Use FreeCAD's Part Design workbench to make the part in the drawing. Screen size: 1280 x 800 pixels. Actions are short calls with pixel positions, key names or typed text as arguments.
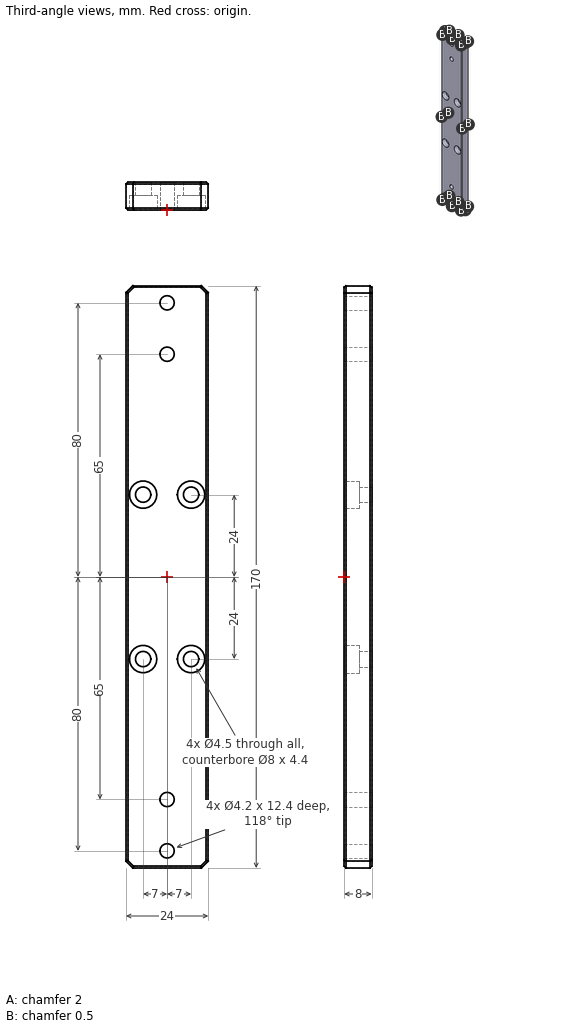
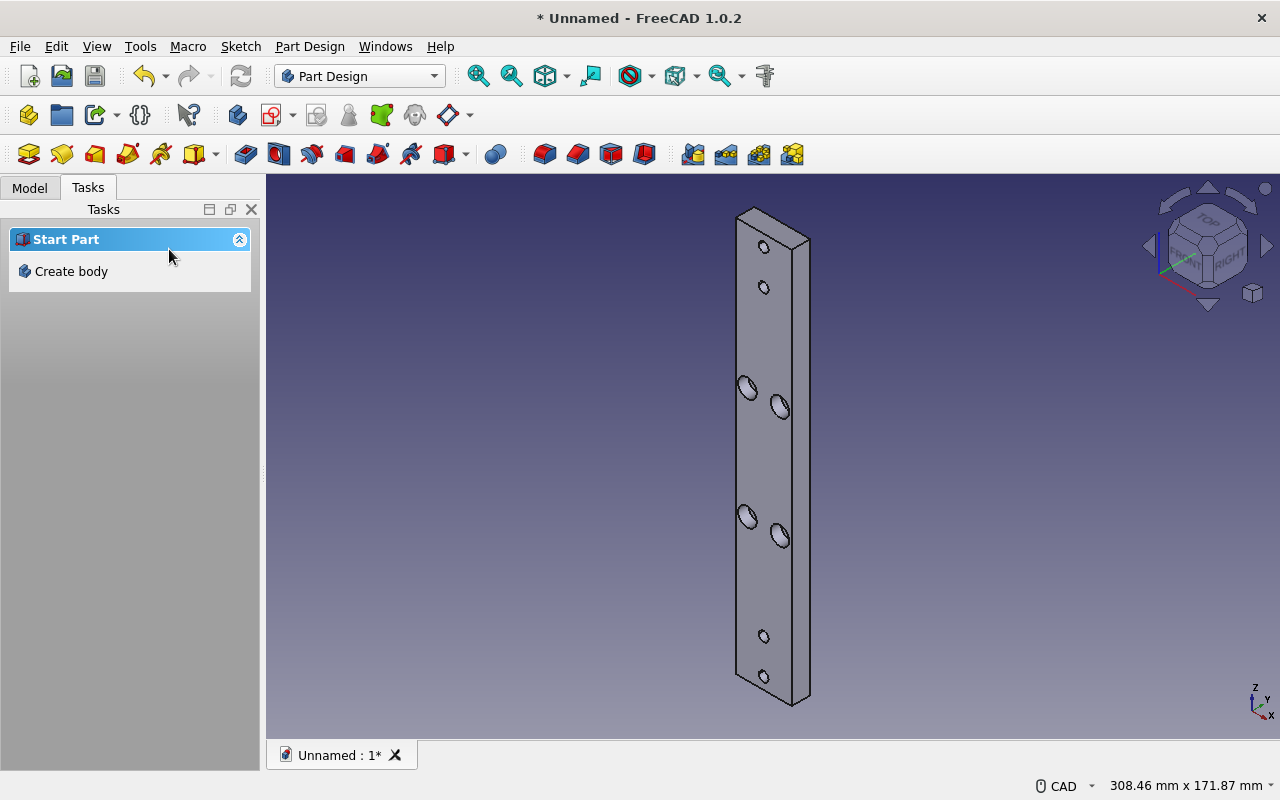
click(801, 243)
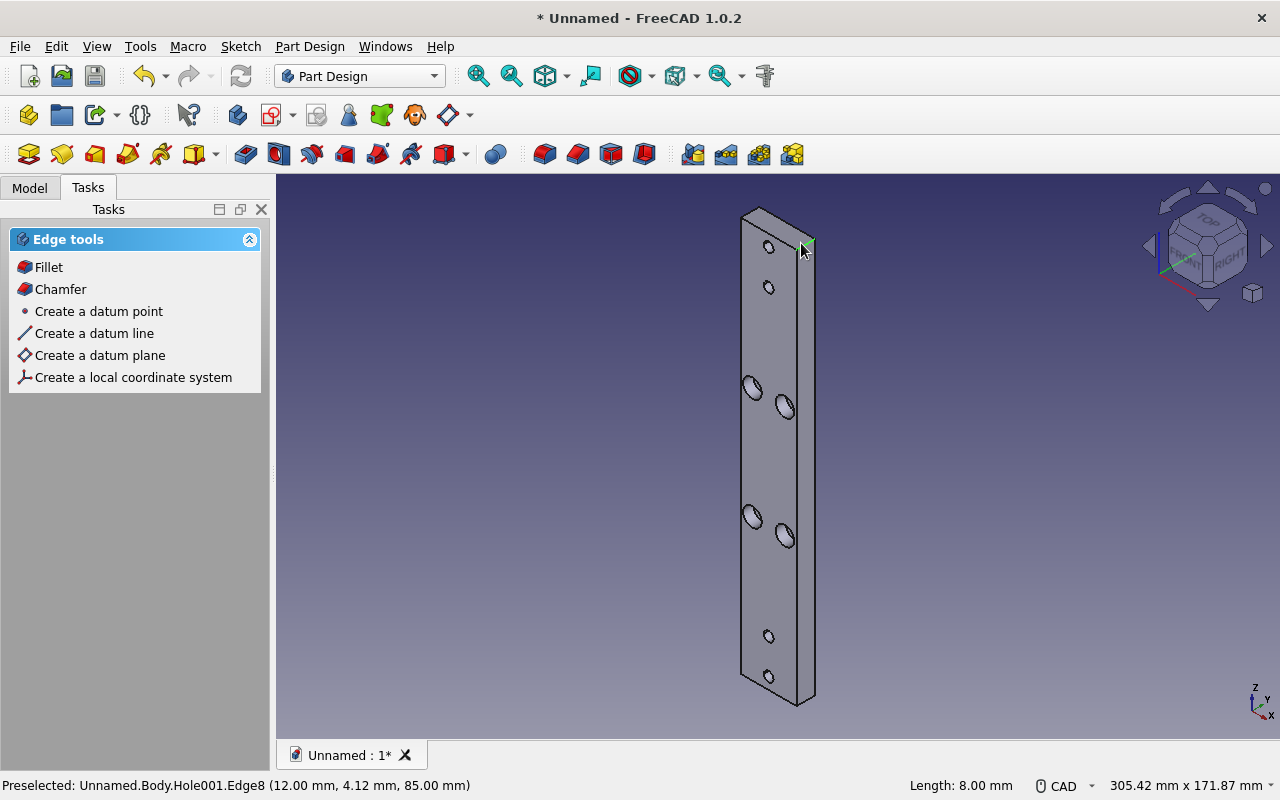
key(2)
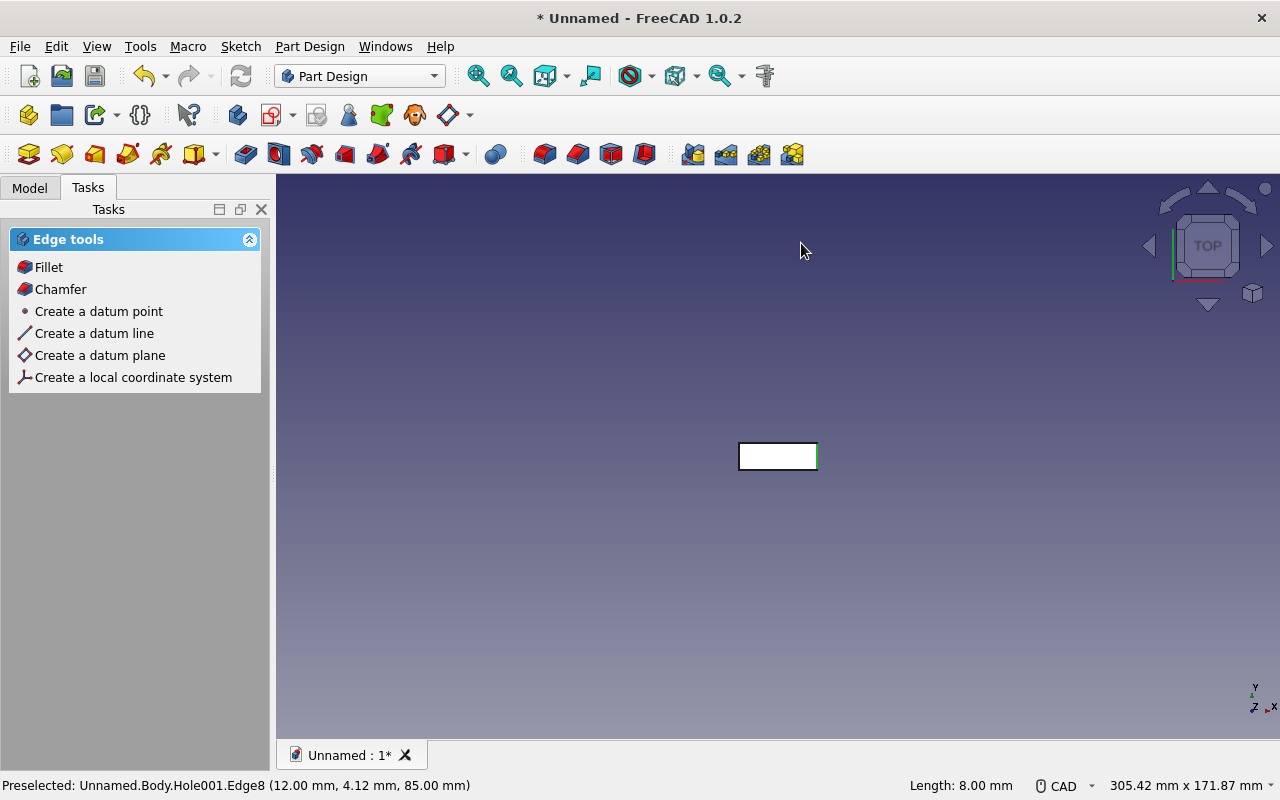
key(v)
key(f)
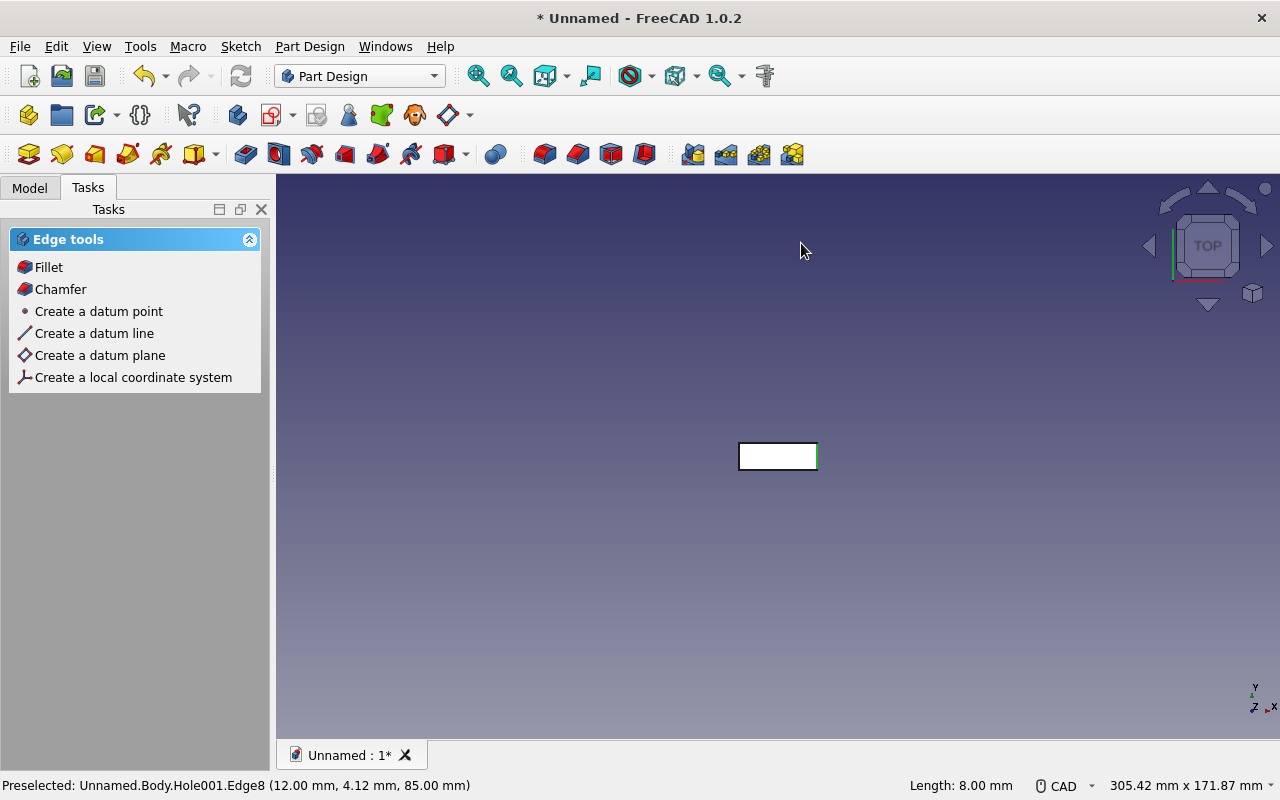
click(739, 455, ctrl)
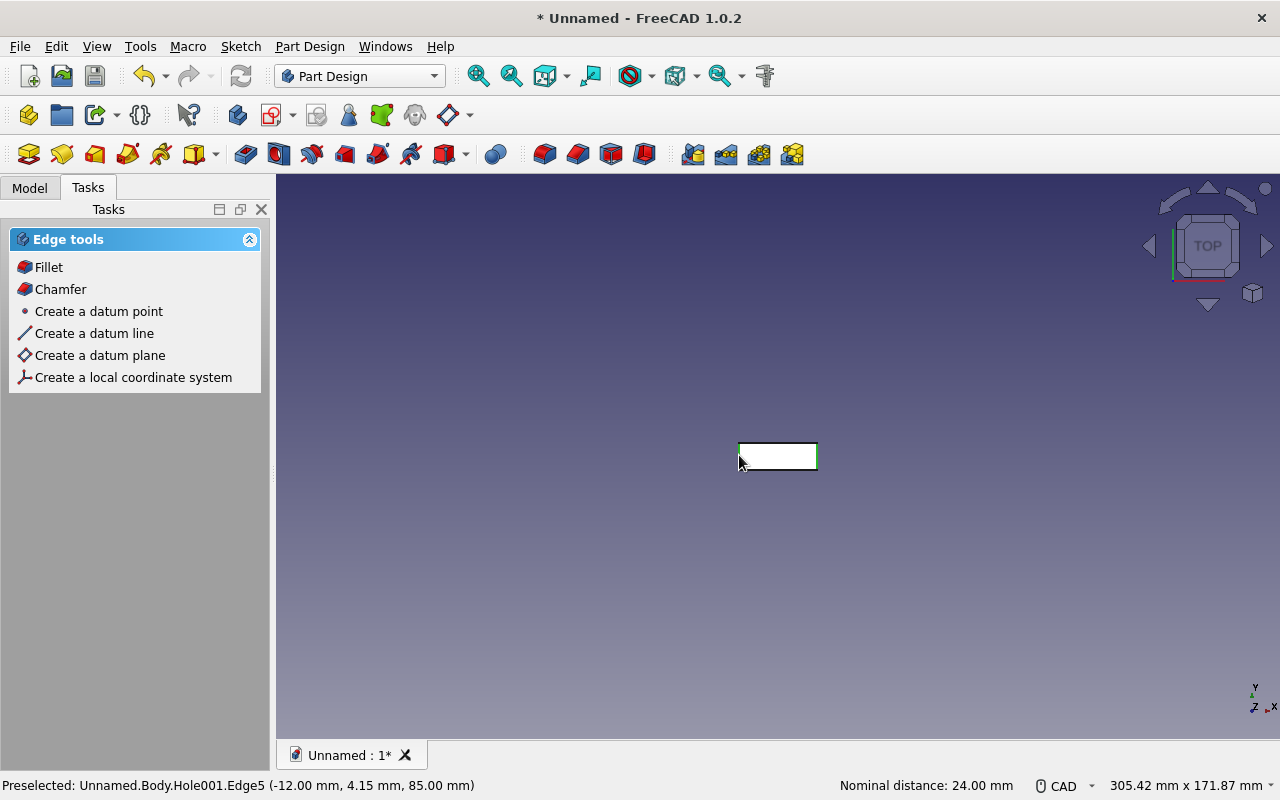
key(1)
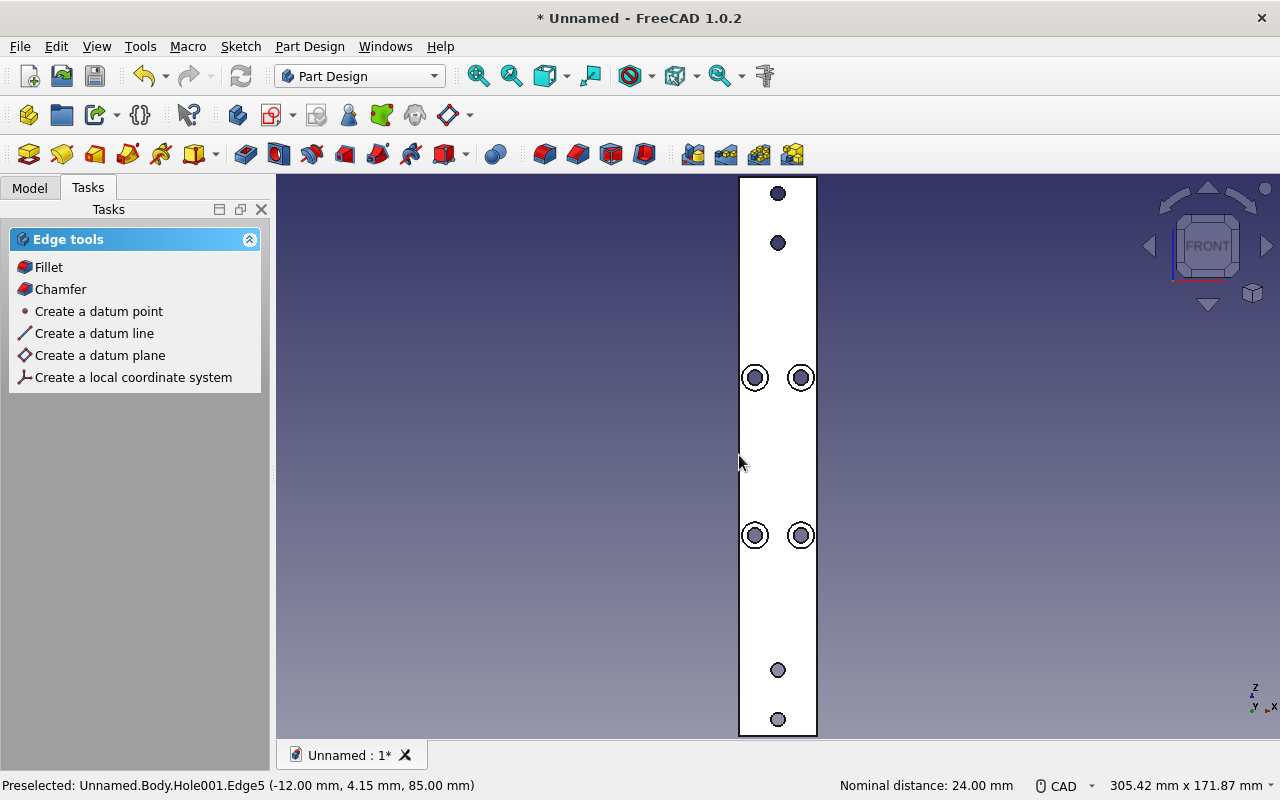
key(3)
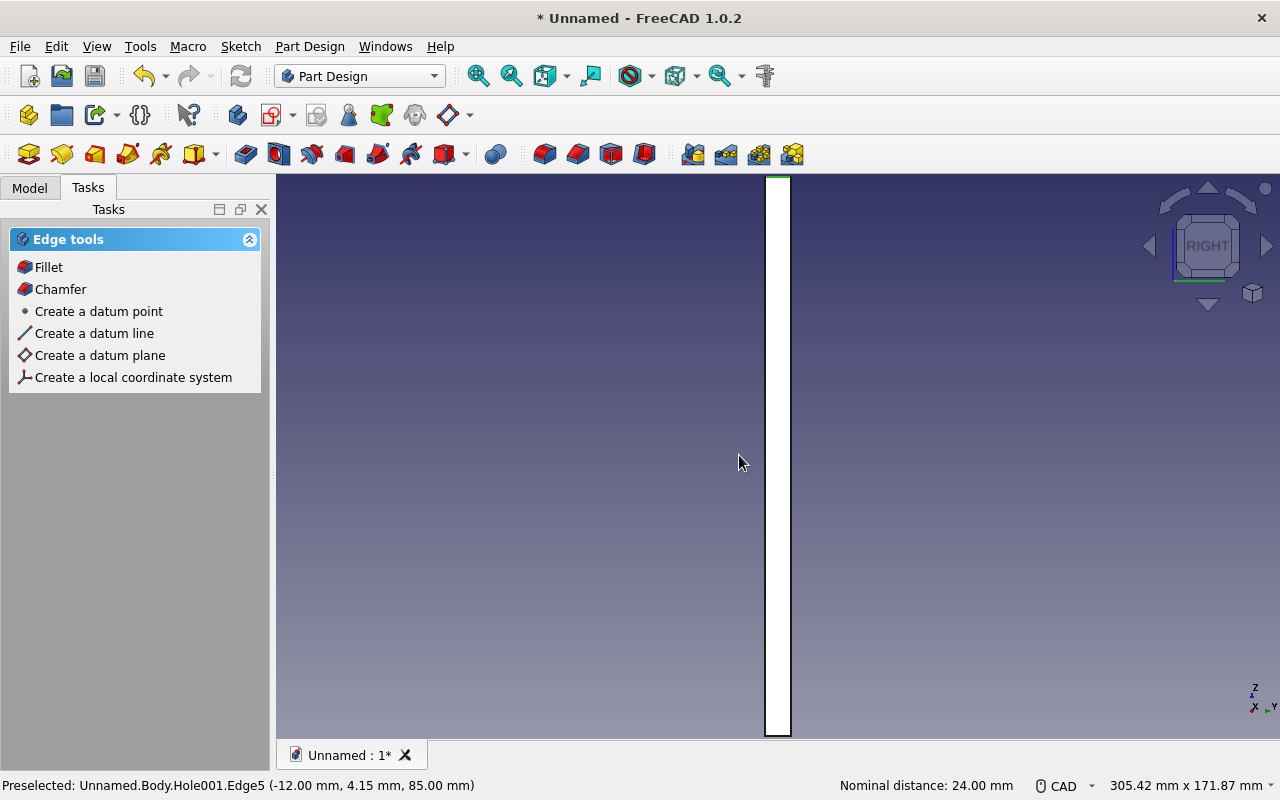
key(5)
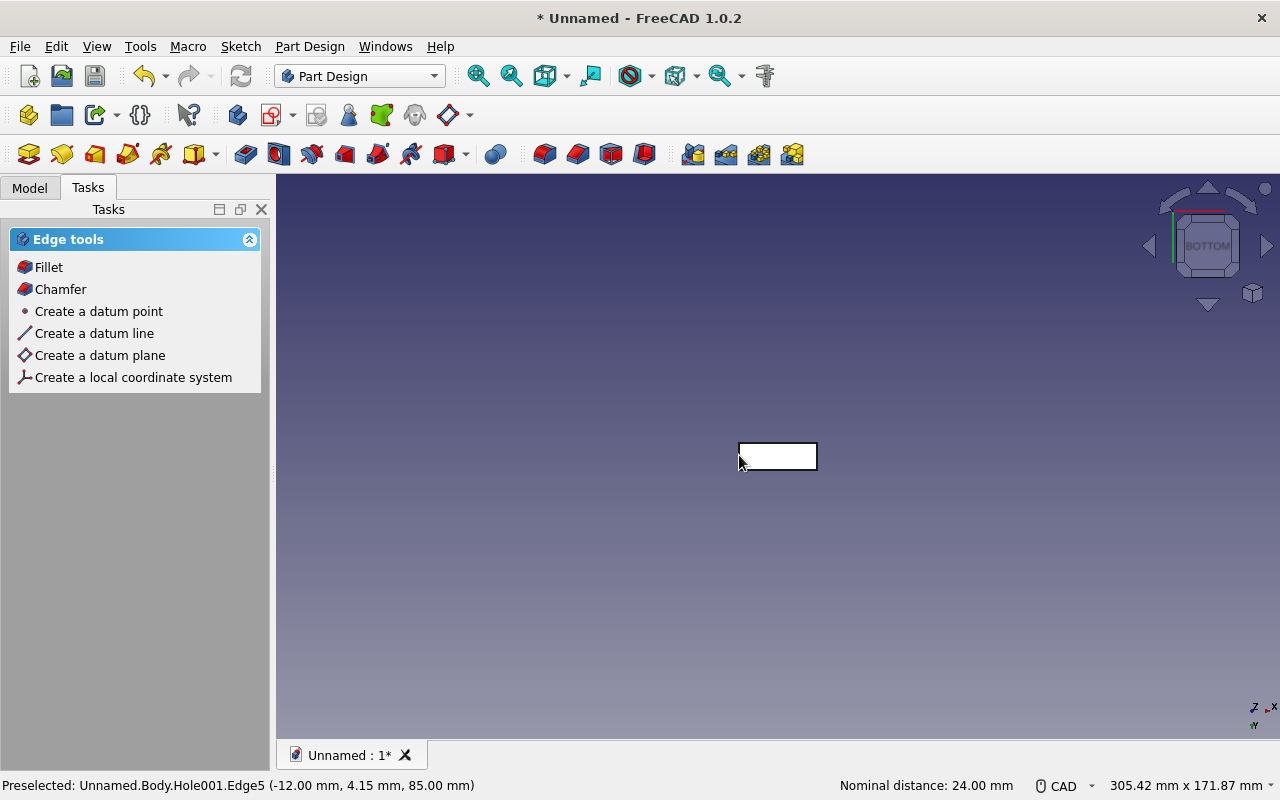
click(479, 76)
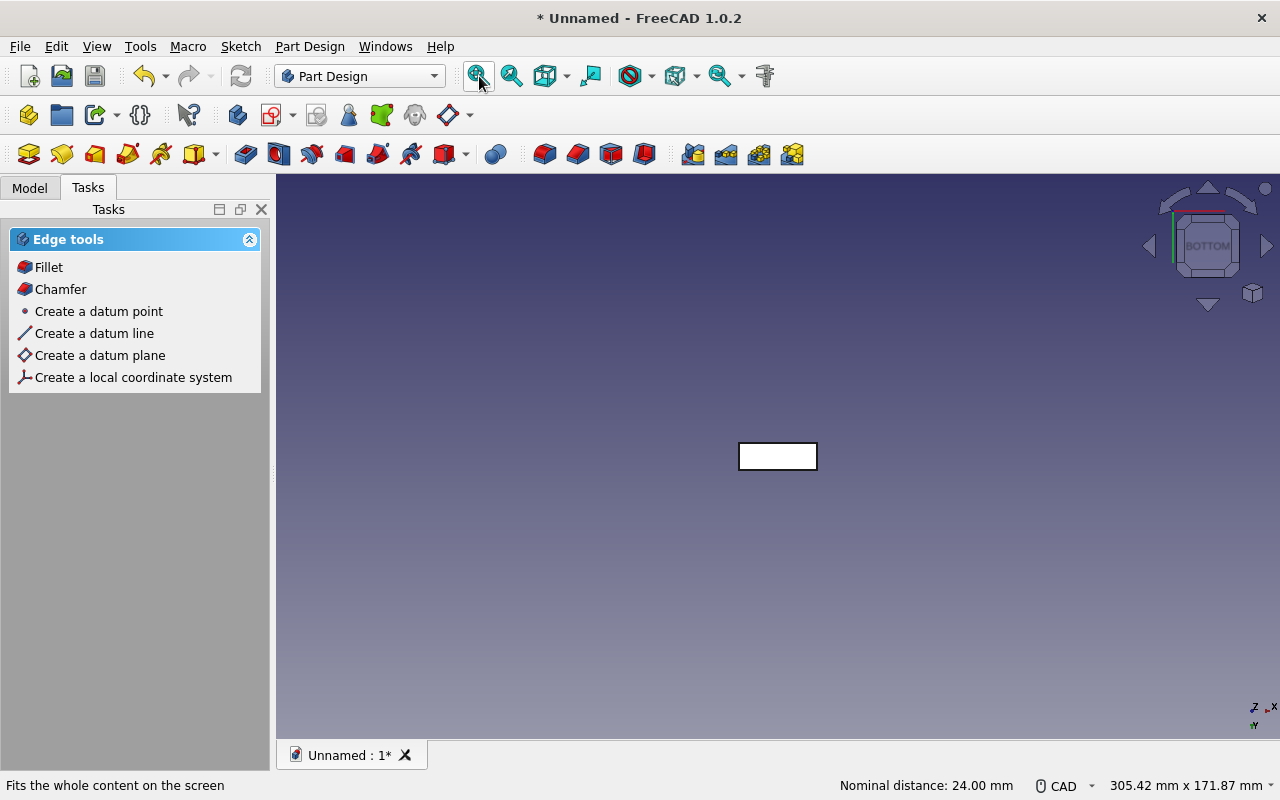
click(739, 455, ctrl)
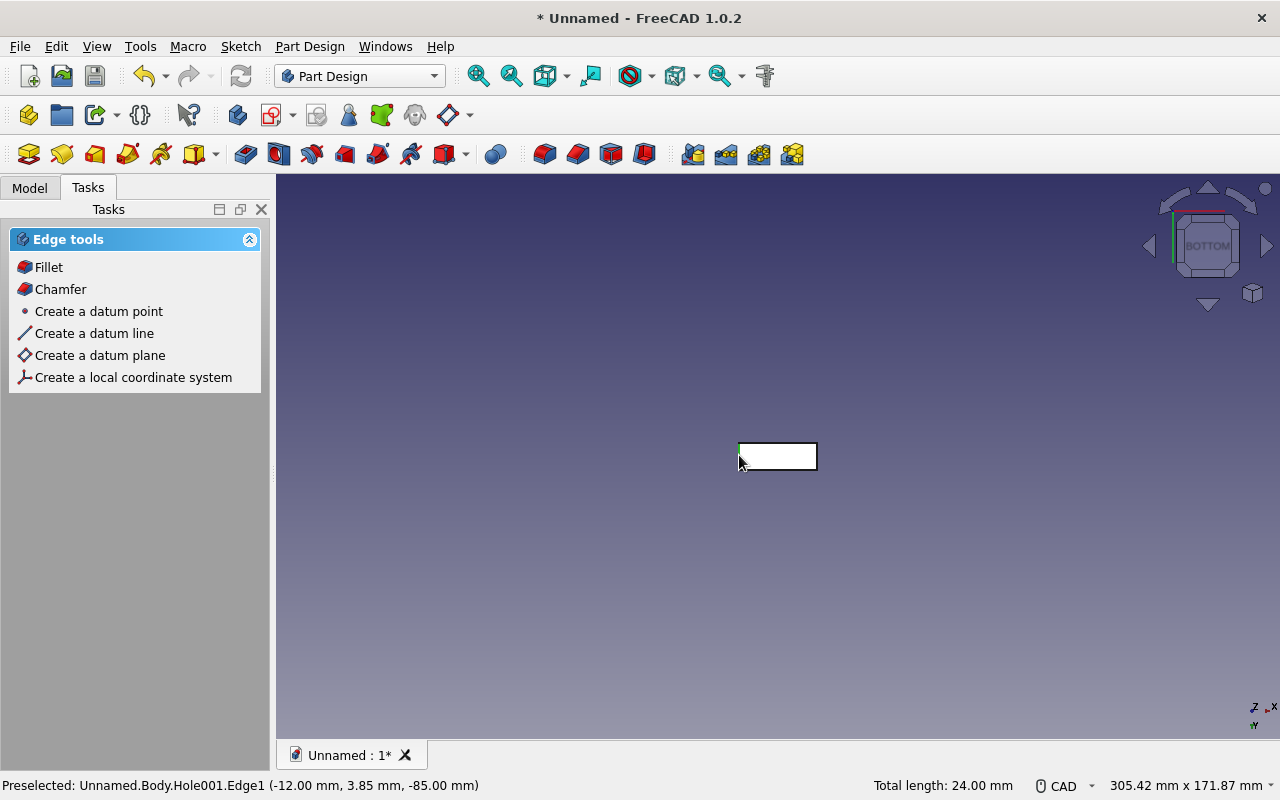
click(817, 455, ctrl)